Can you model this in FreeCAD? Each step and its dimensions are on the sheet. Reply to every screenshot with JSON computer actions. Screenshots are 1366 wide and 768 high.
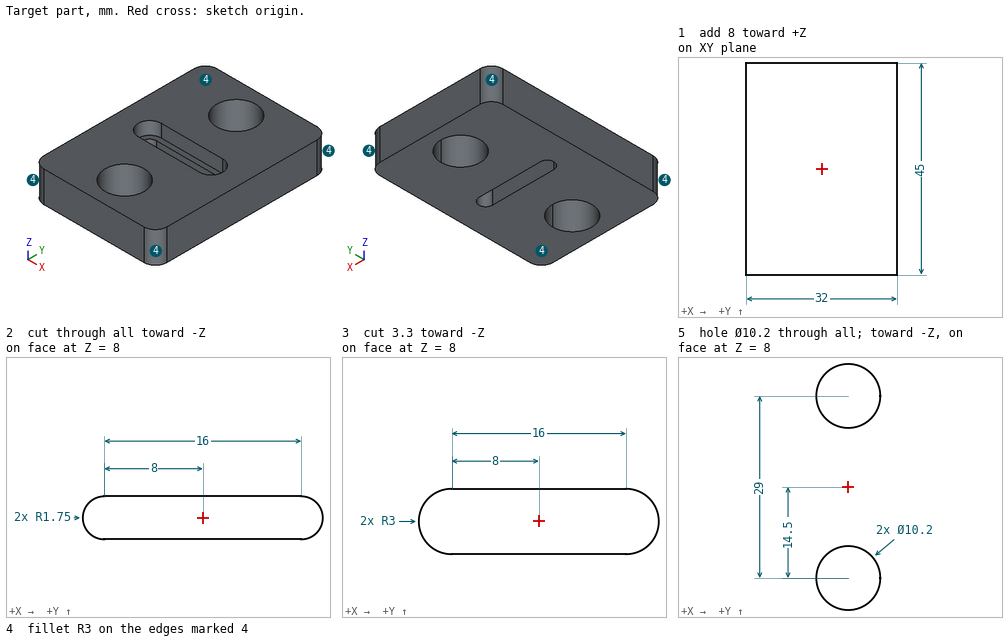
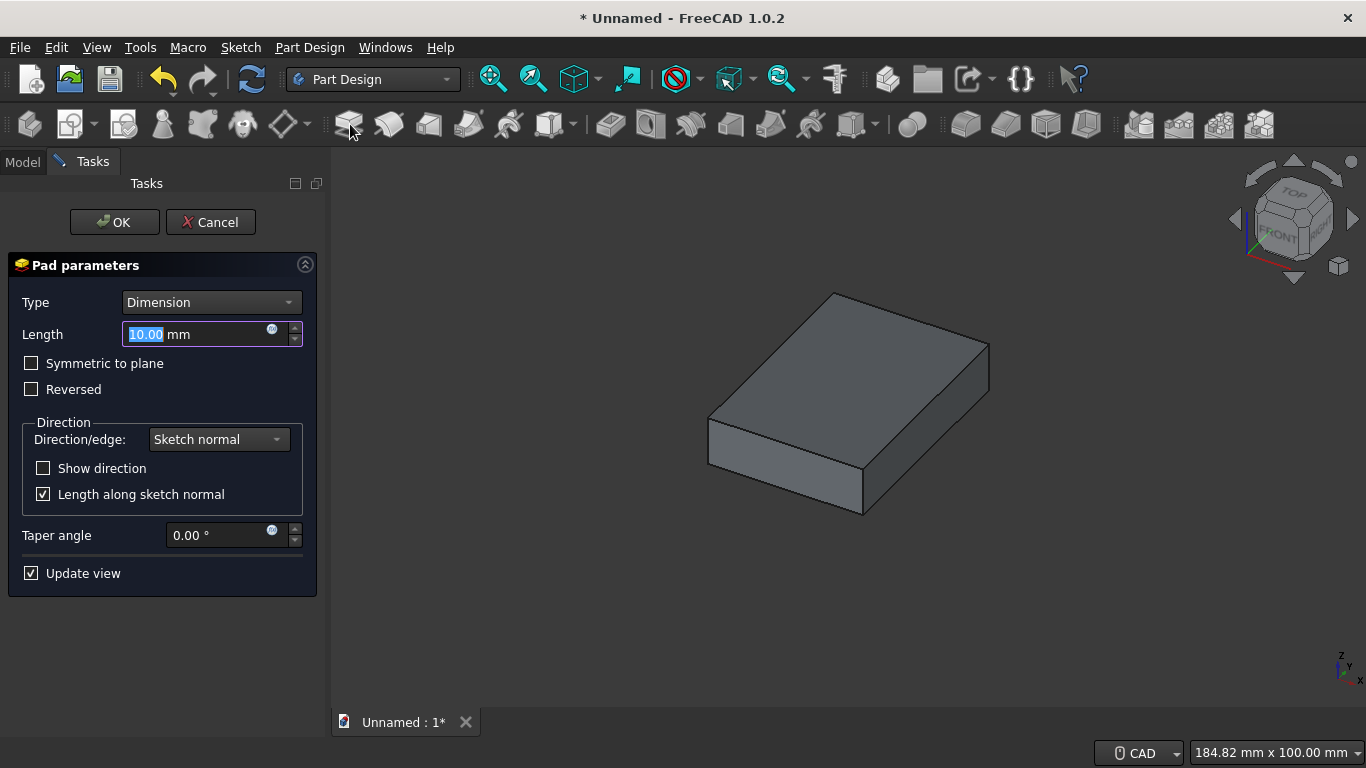
{"action": "type", "text": "8"}
{"action": "key", "text": "Tab"}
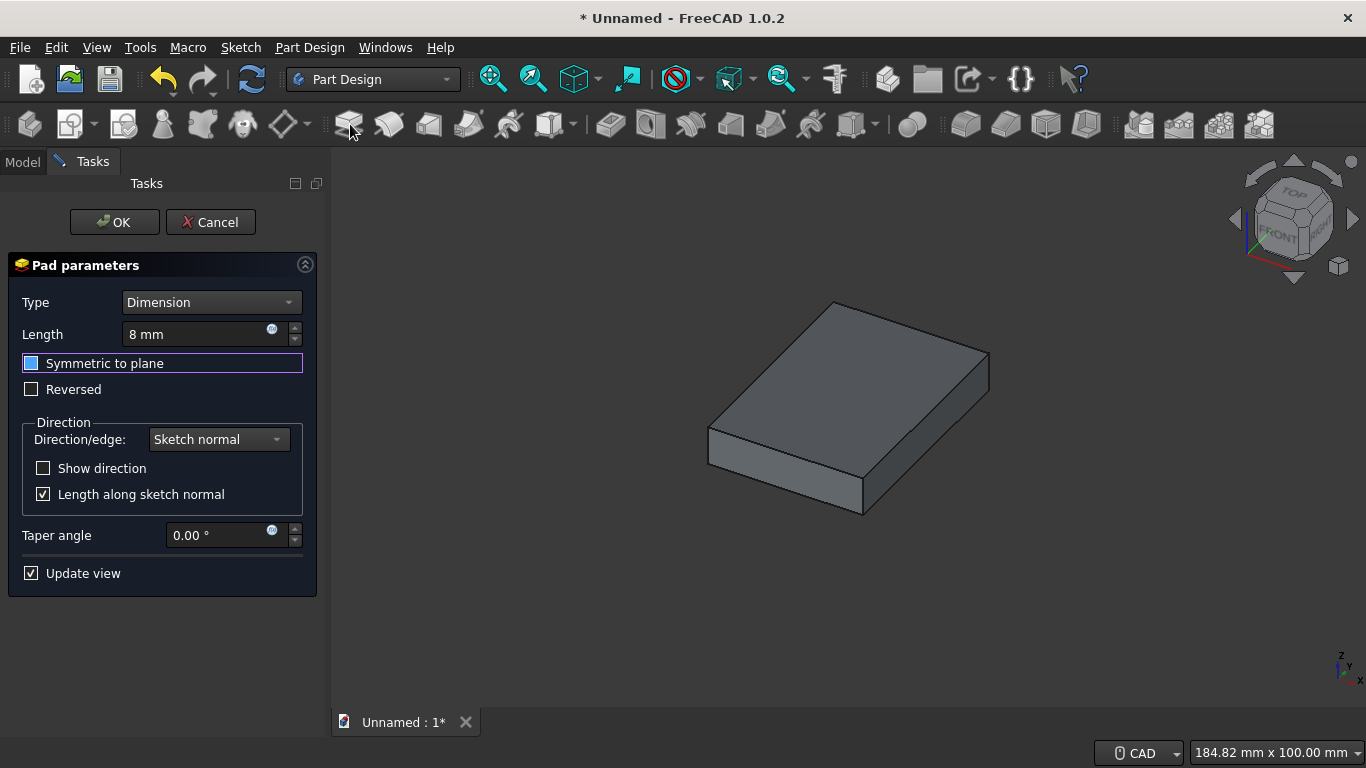
{"action": "left_click", "coordinate": [115, 222]}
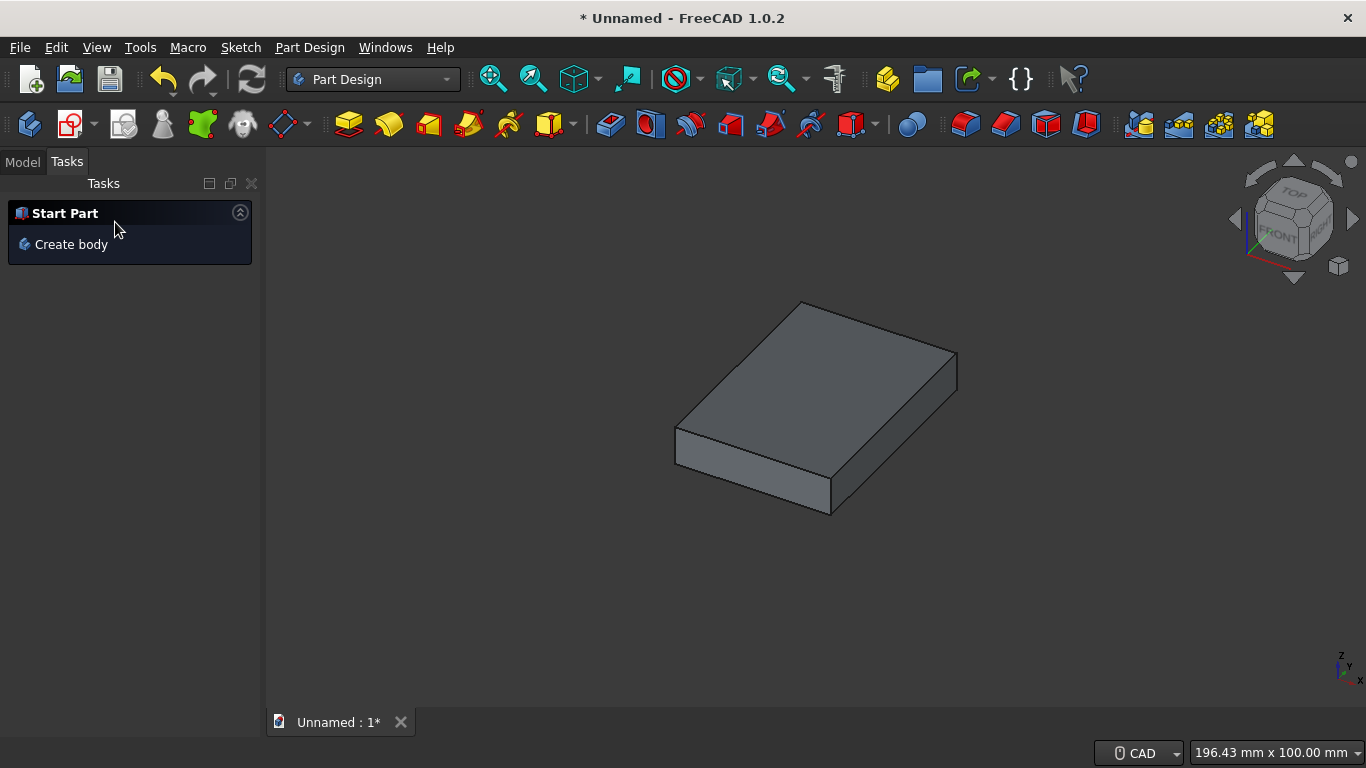
{"action": "key", "text": "v f"}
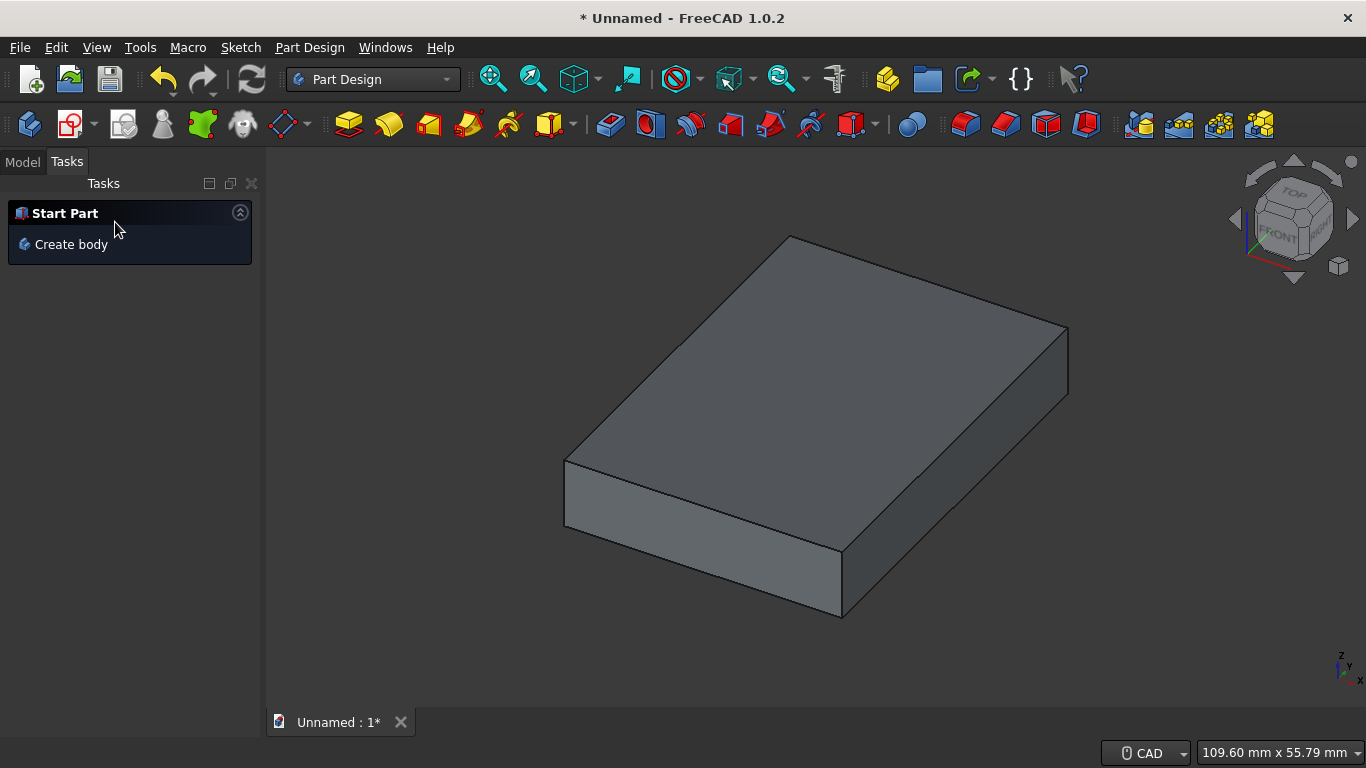
{"action": "left_click", "coordinate": [848, 361]}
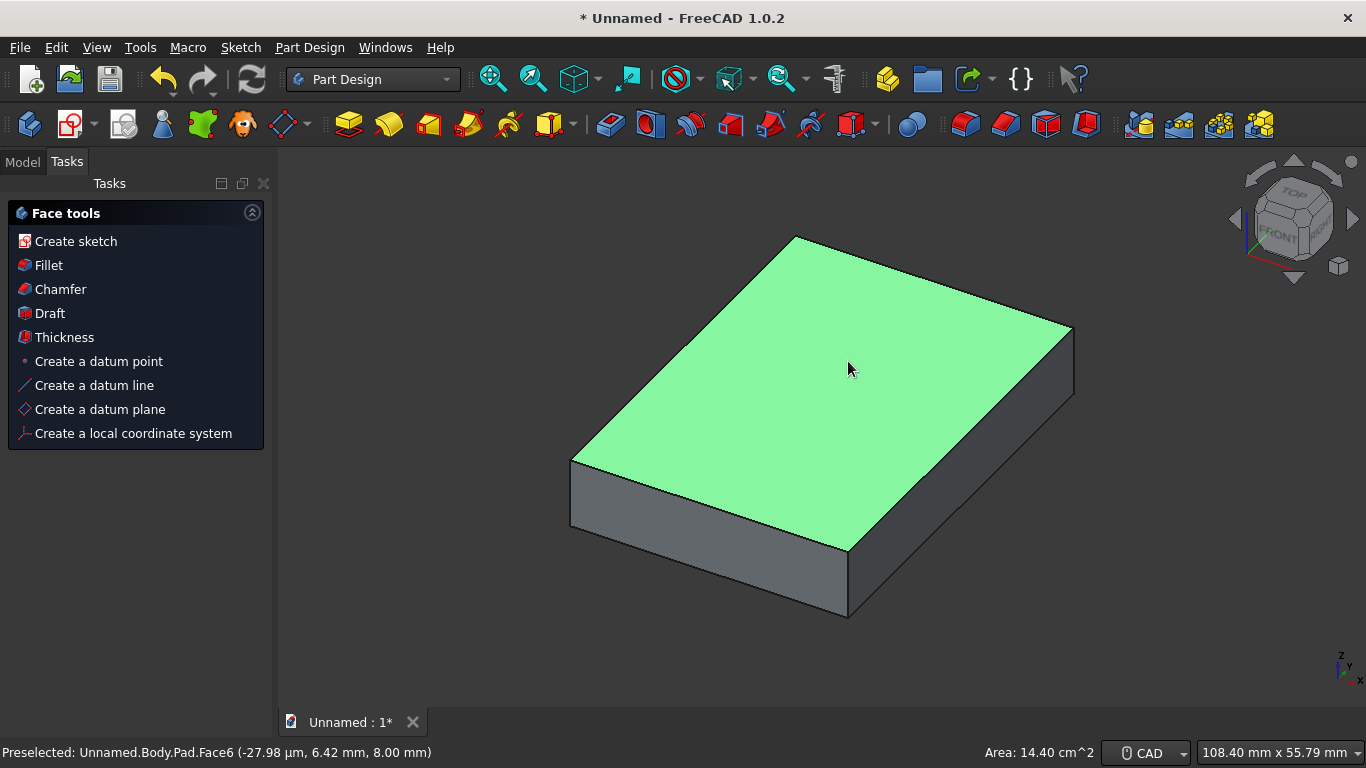
{"action": "left_click", "coordinate": [70, 124]}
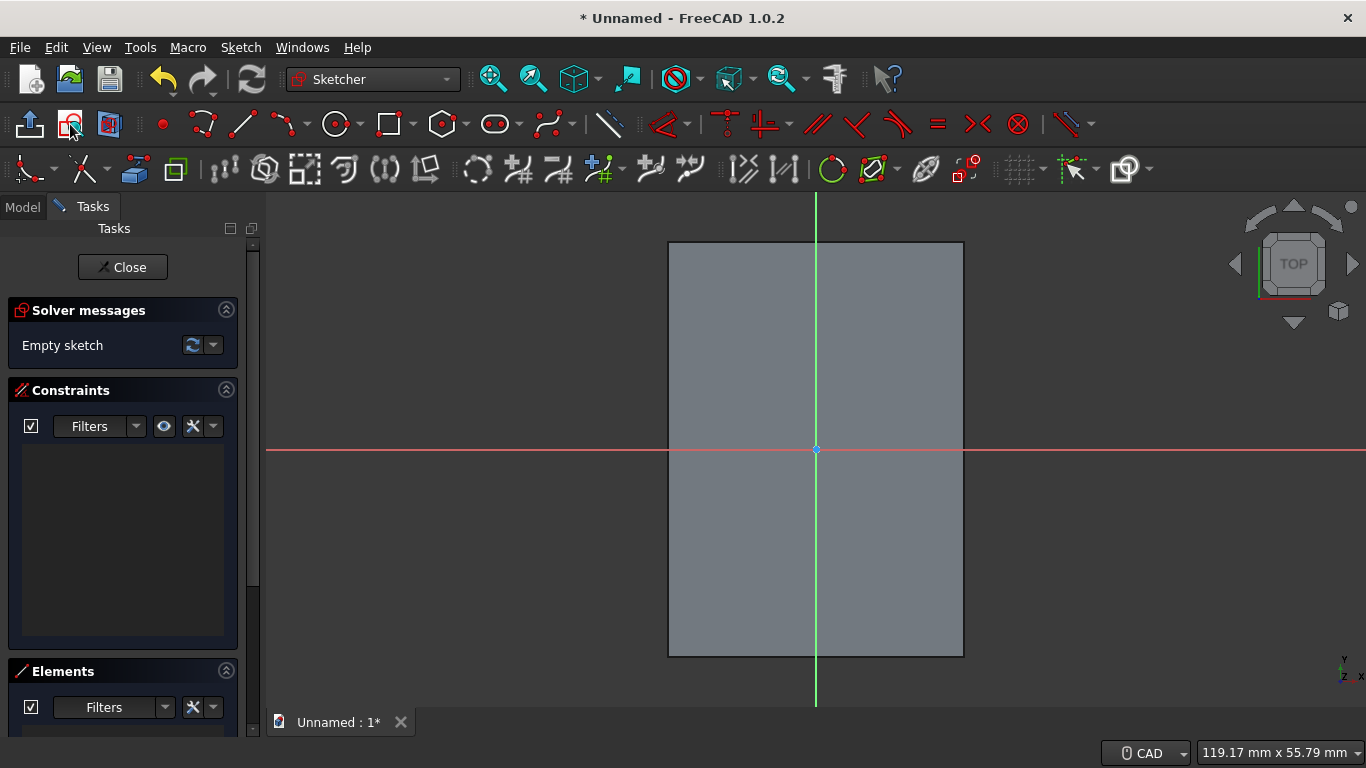
{"action": "scroll", "coordinate": [846, 449], "scroll_direction": "up", "scroll_amount": 6}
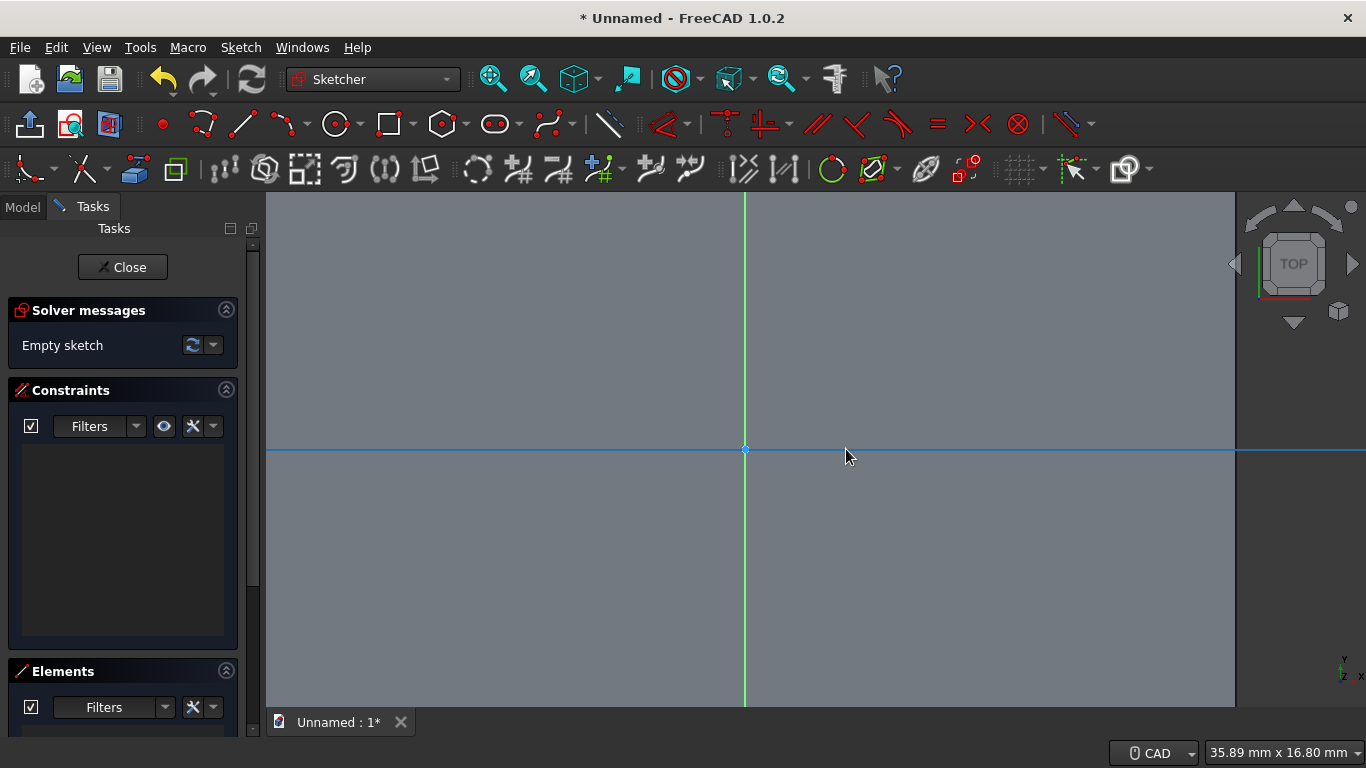
{"action": "key", "text": "g s"}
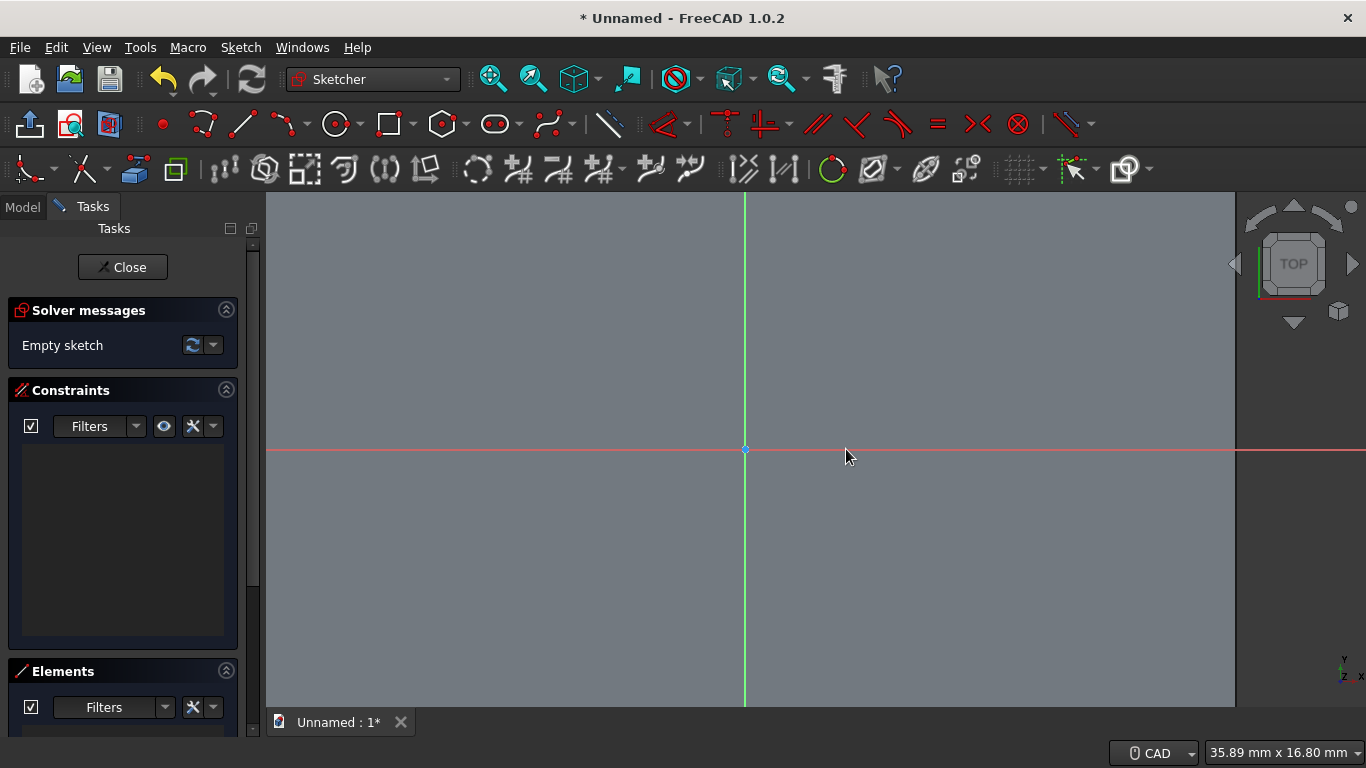
{"action": "left_click", "coordinate": [500, 450]}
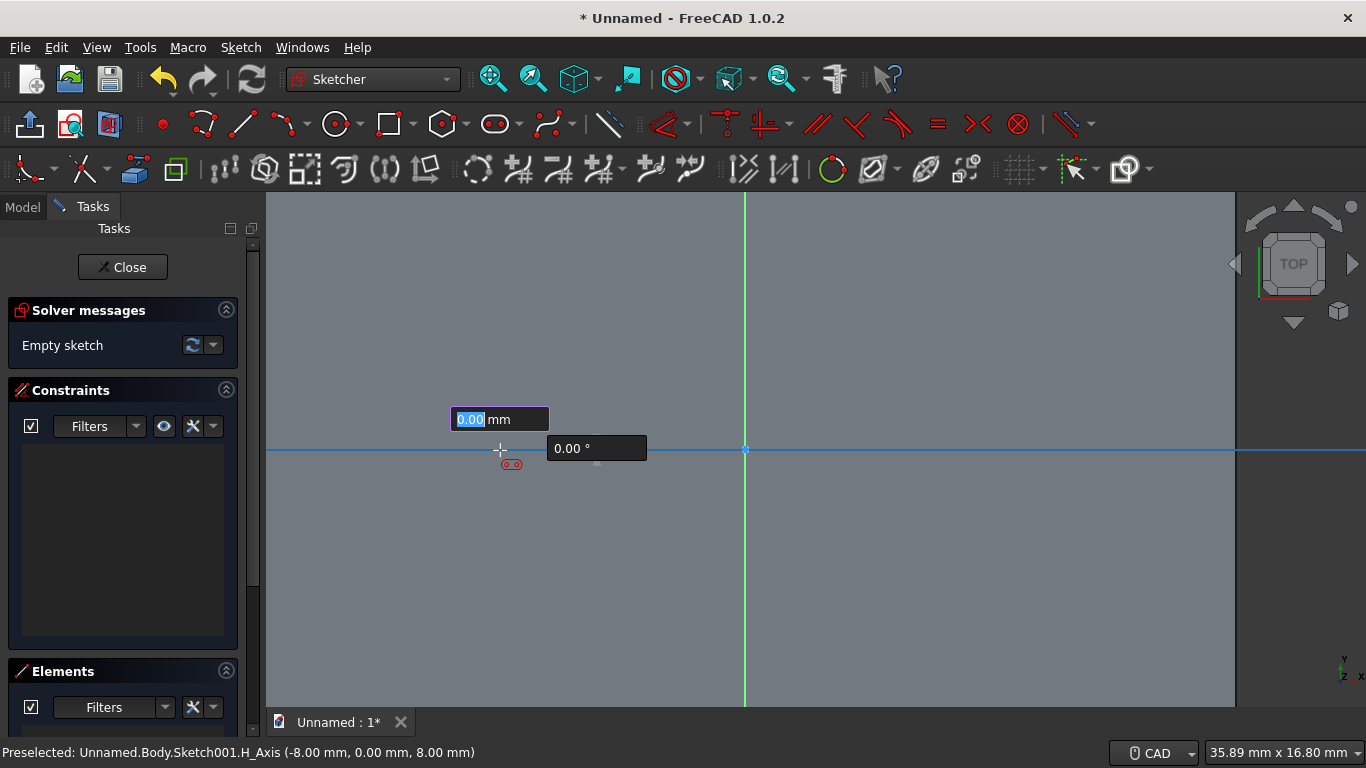
{"action": "left_click", "coordinate": [990, 440]}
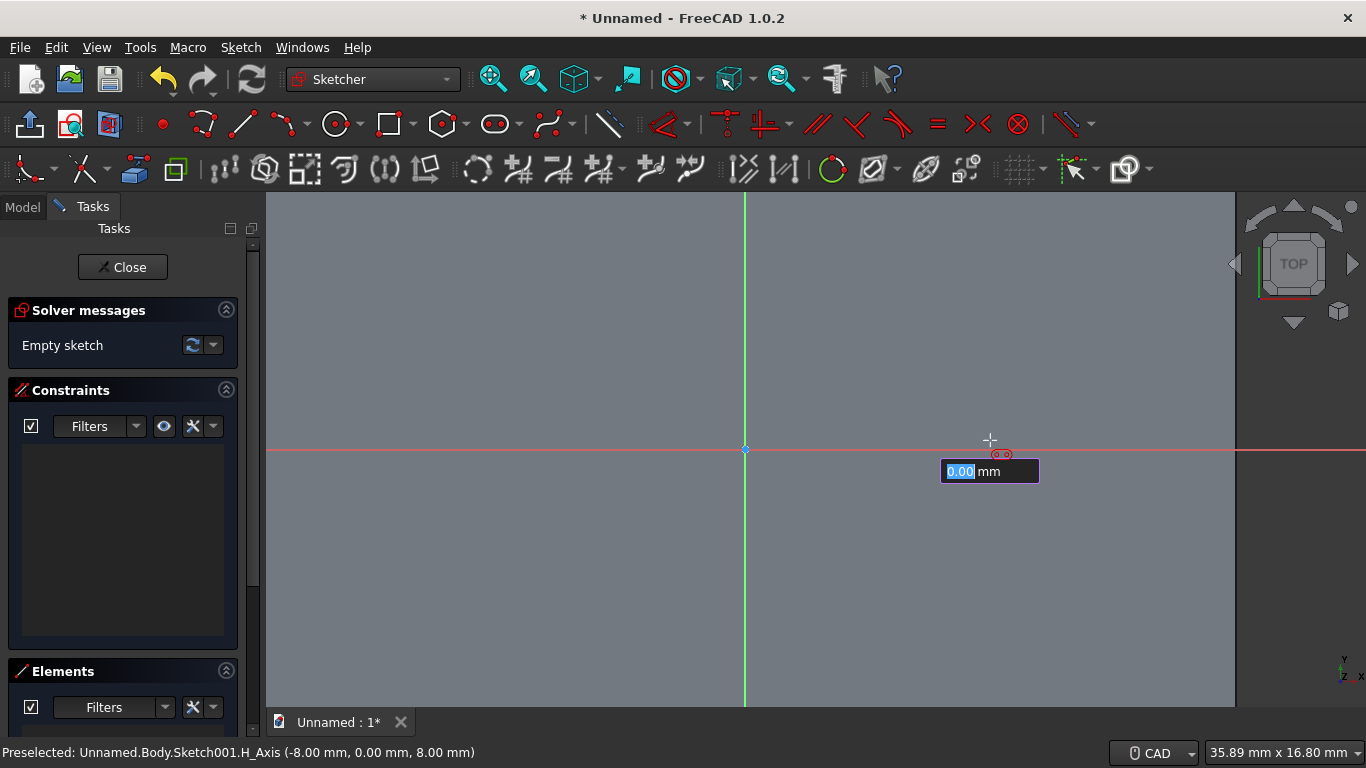
{"action": "left_click", "coordinate": [819, 396]}
{"action": "key", "text": "Escape"}